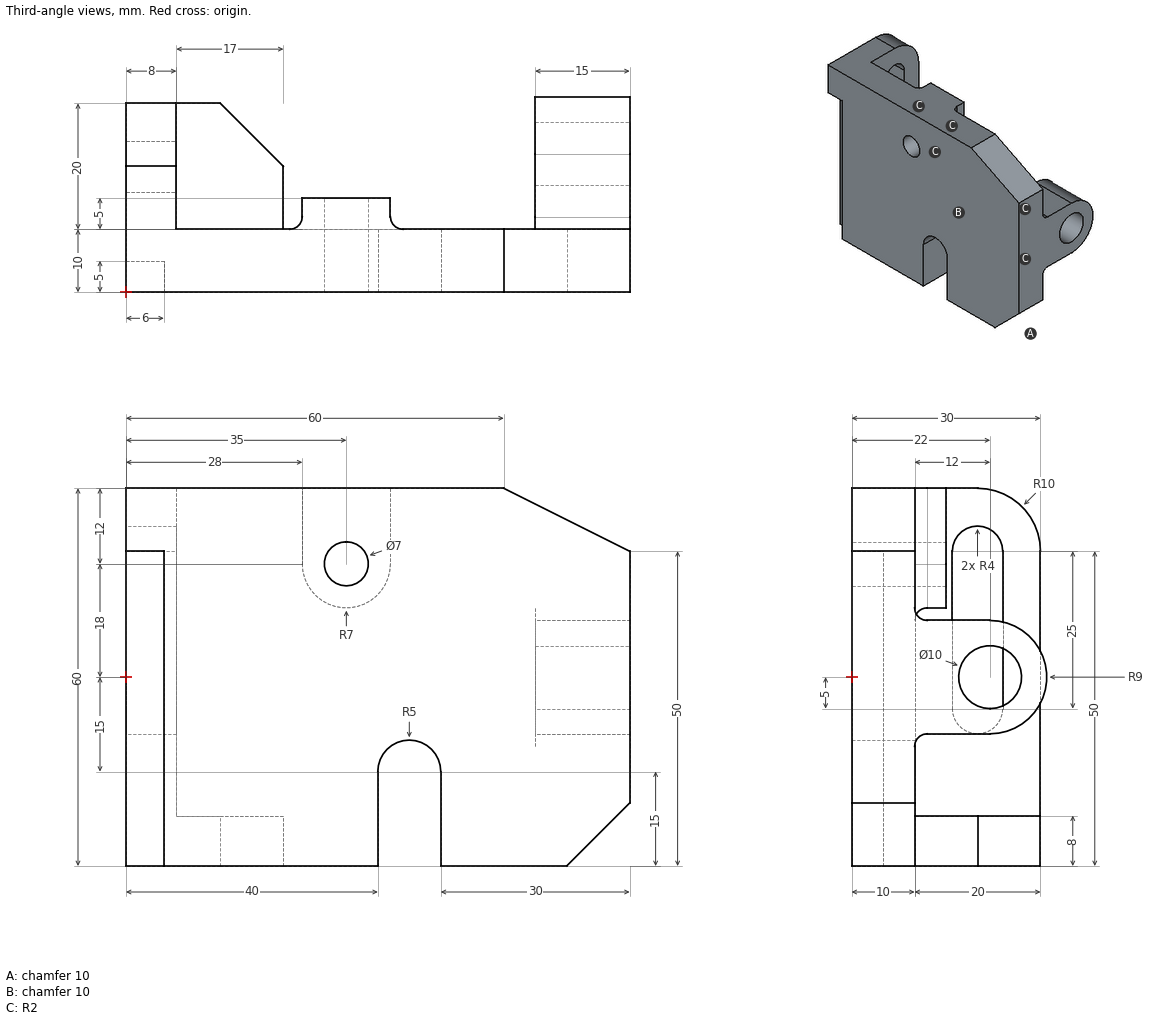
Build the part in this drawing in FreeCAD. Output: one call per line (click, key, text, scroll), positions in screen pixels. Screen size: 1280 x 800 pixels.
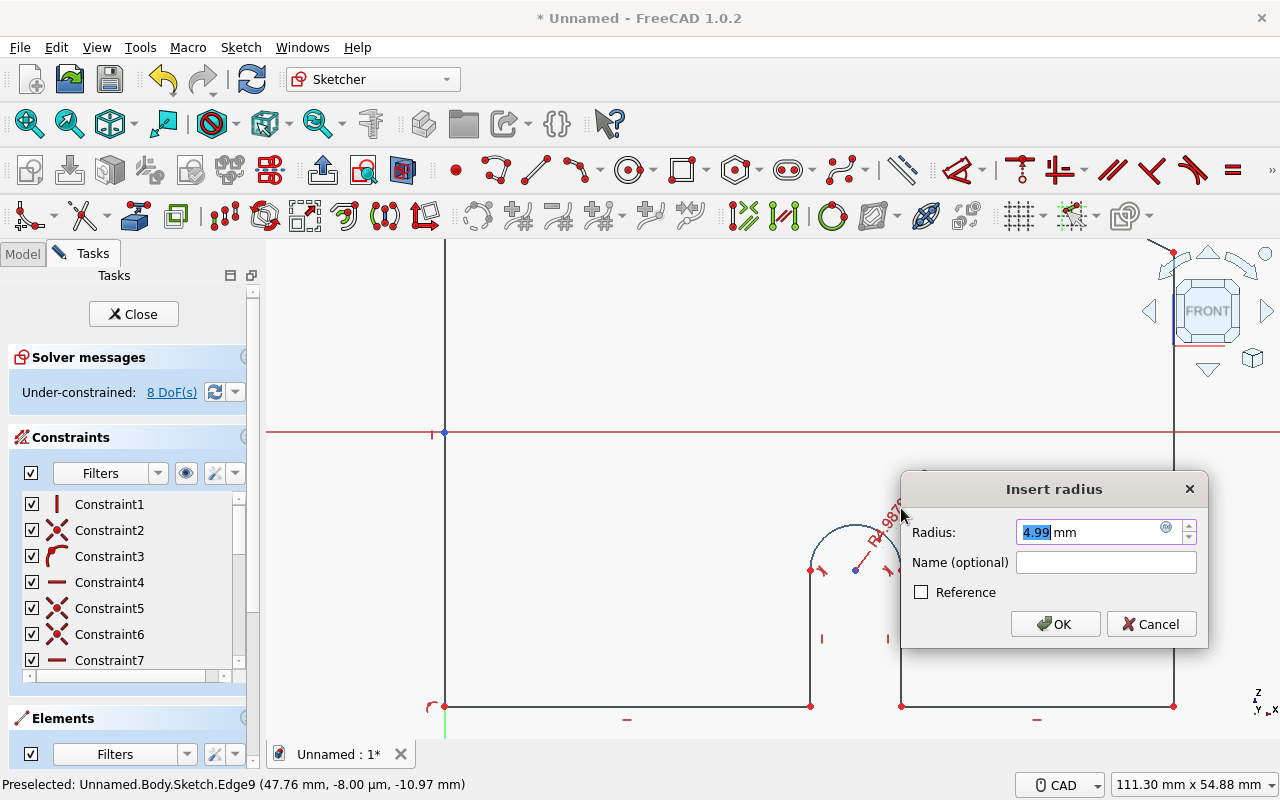
text(5)
key(Return)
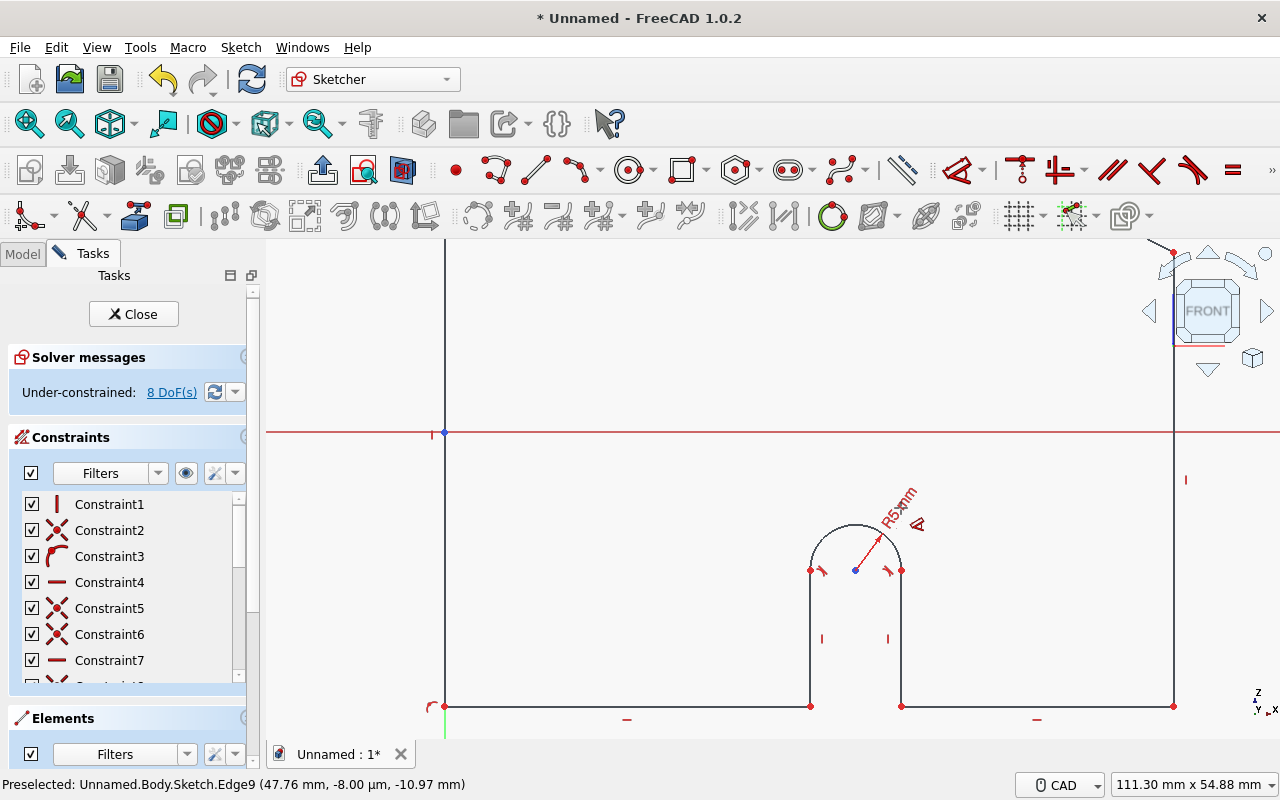
click(810, 611)
click(844, 639)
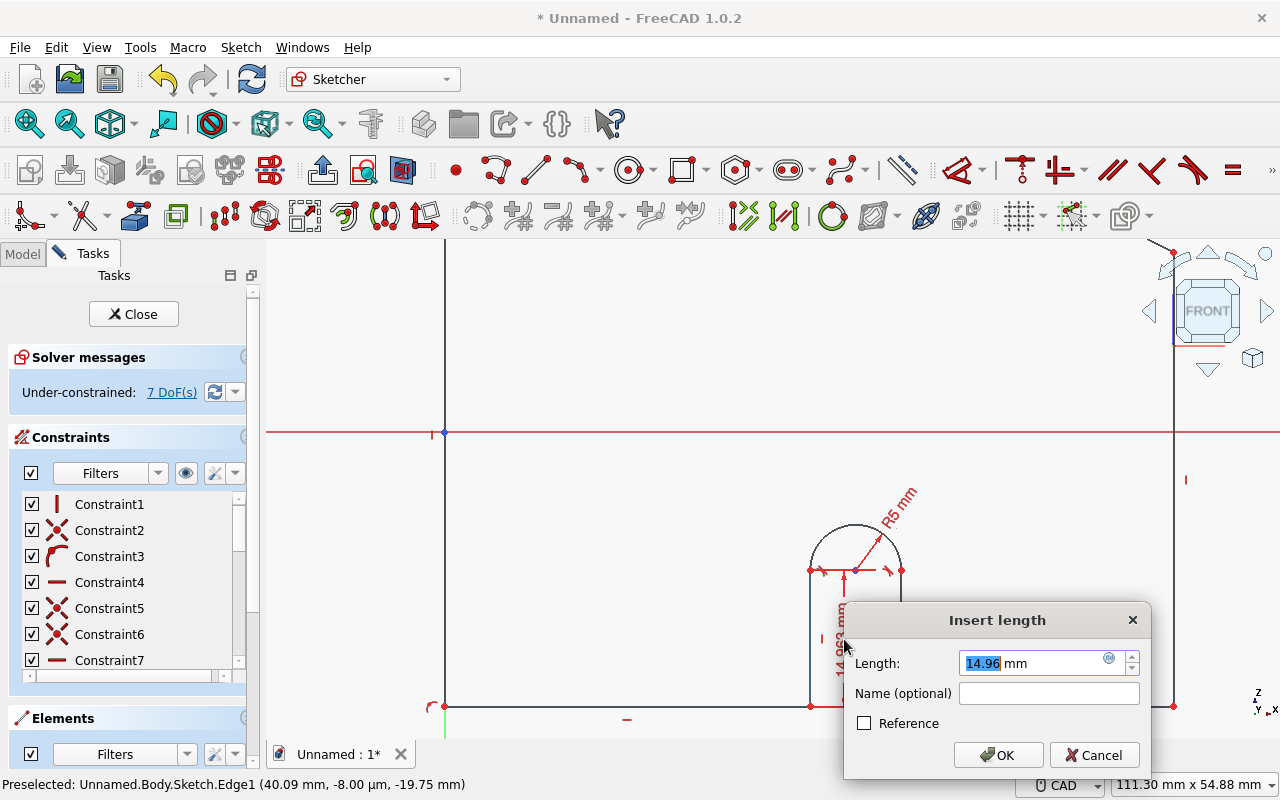
text(15)
key(Return)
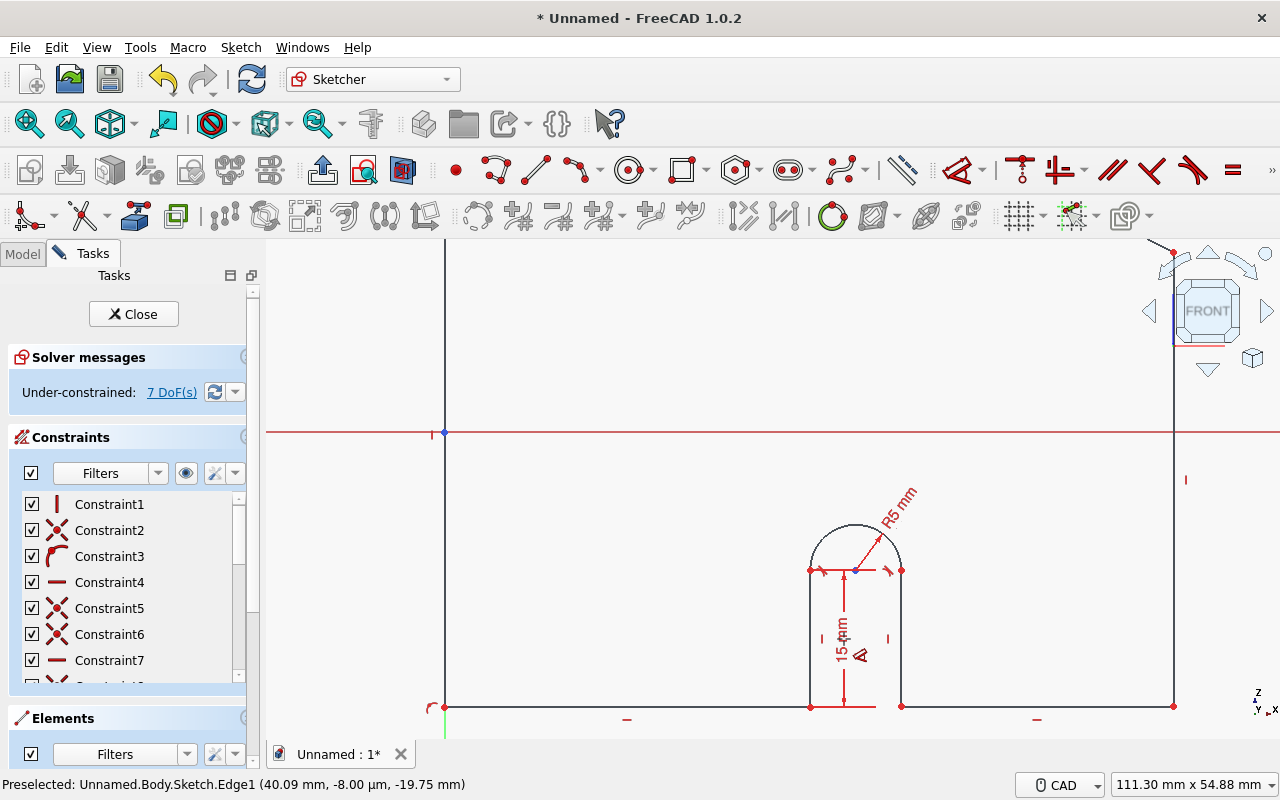
click(701, 707)
click(628, 673)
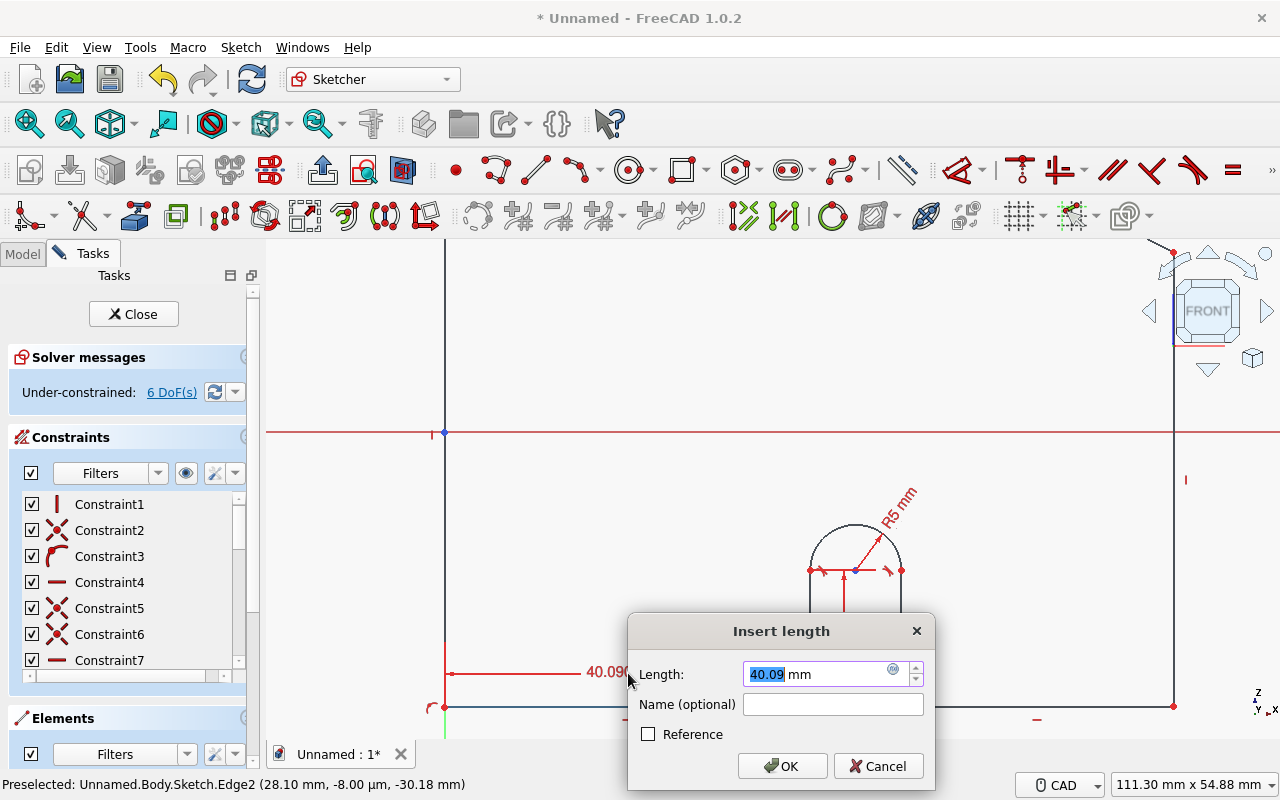
text(40)
key(Return)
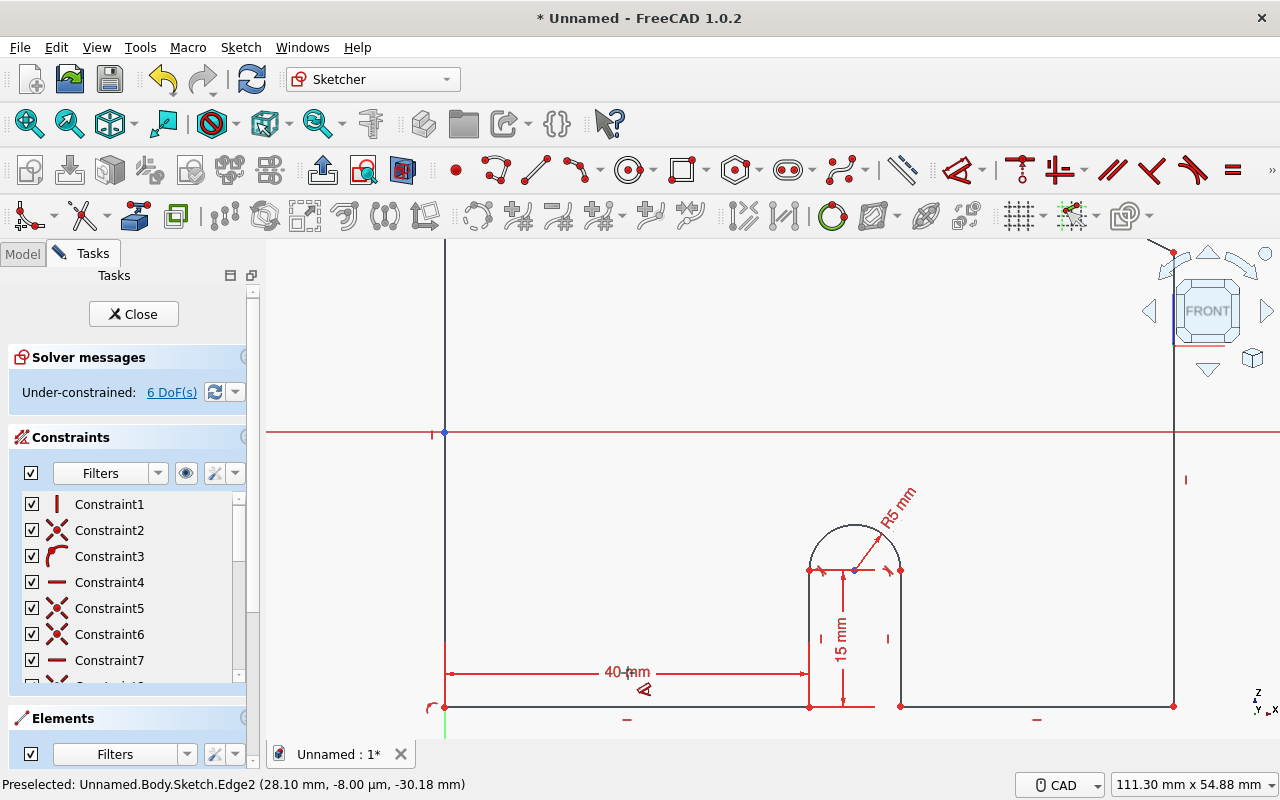
click(445, 543)
click(411, 487)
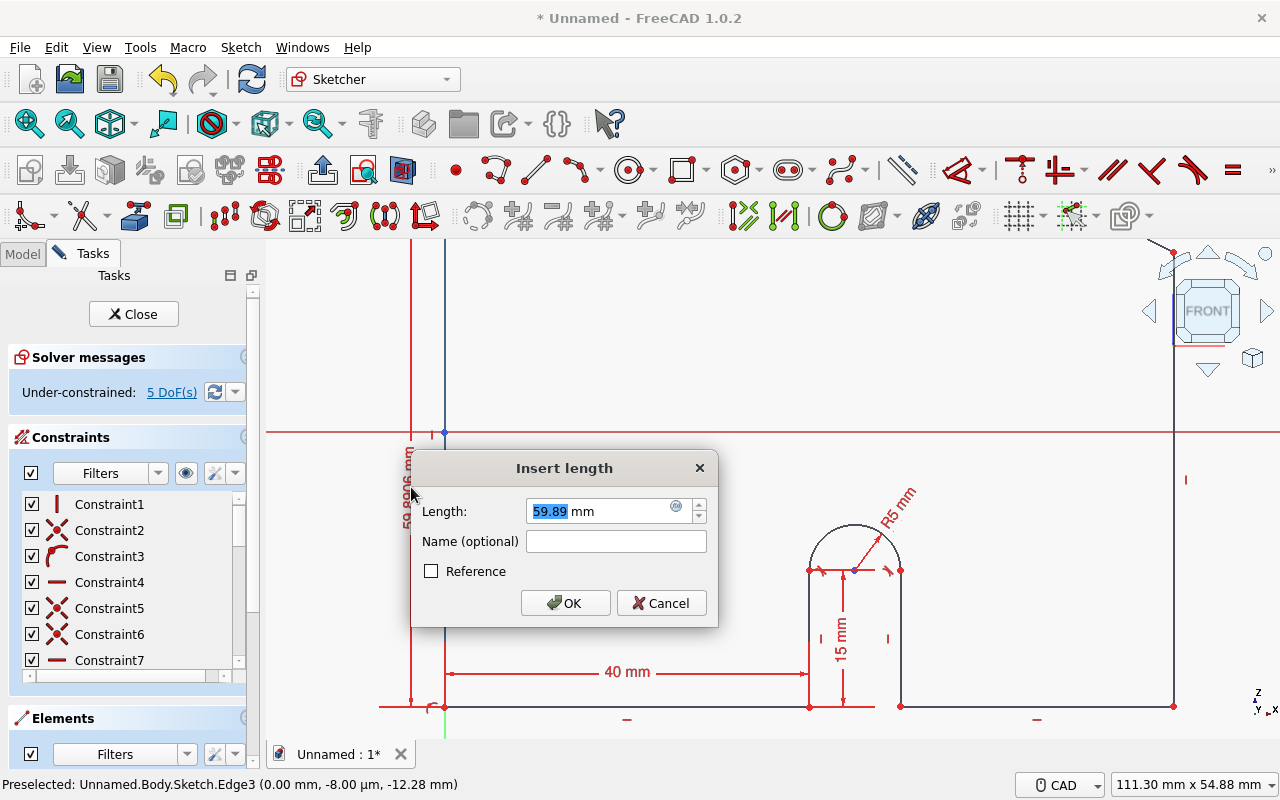
text(60)
key(Return)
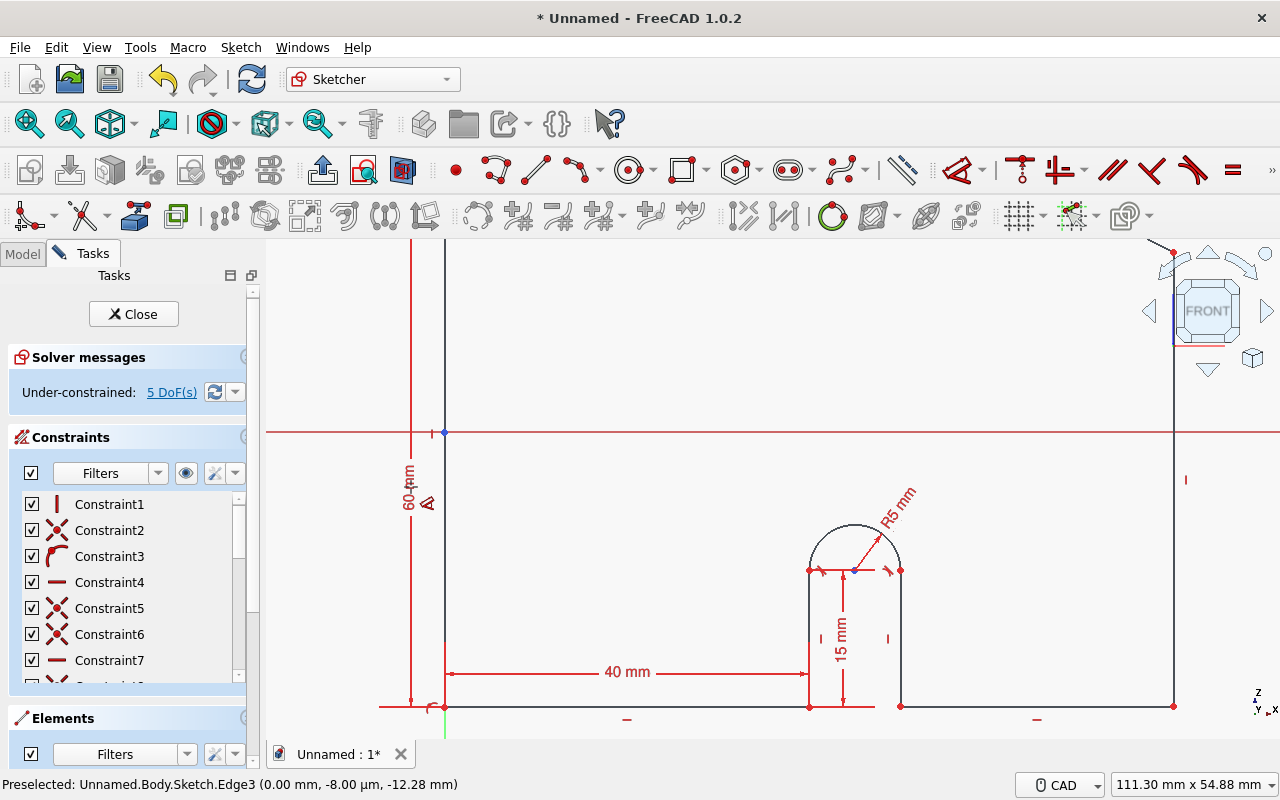
scroll(577, 558, down, 3)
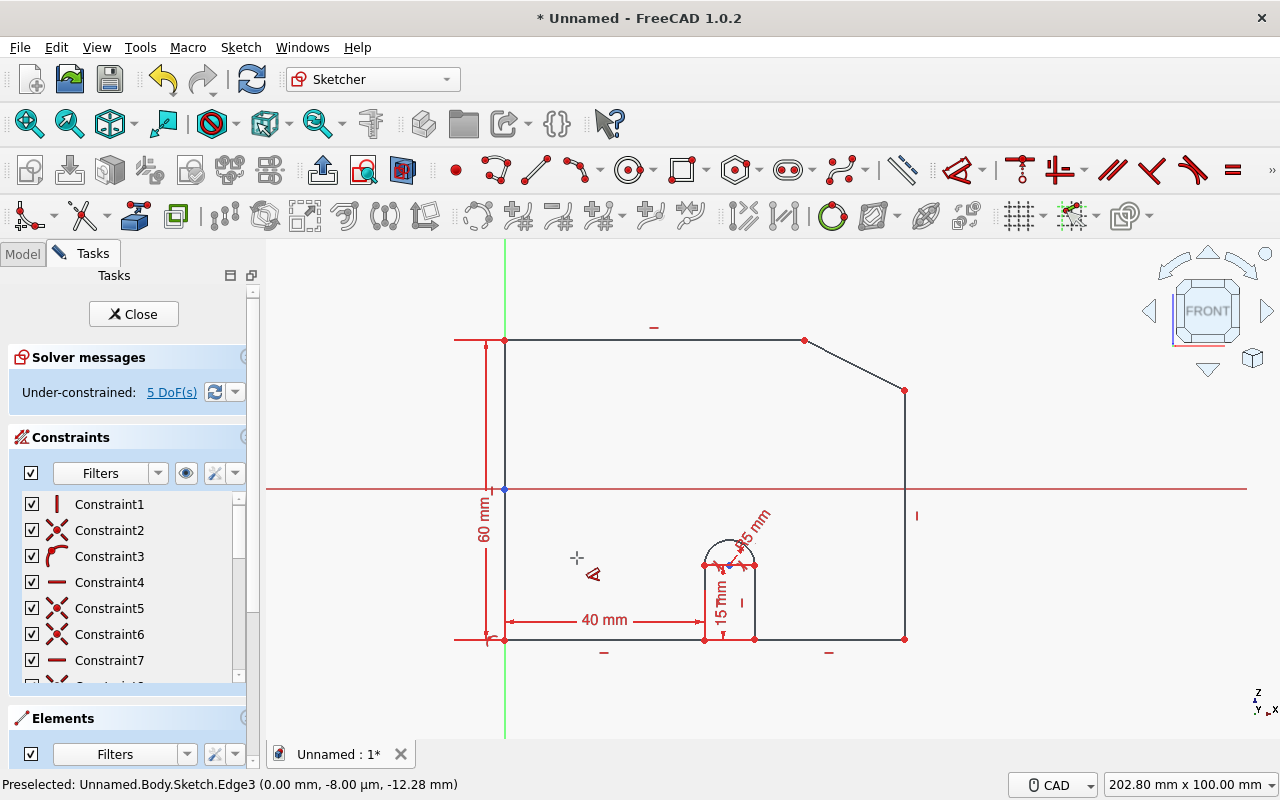
click(595, 340)
click(655, 306)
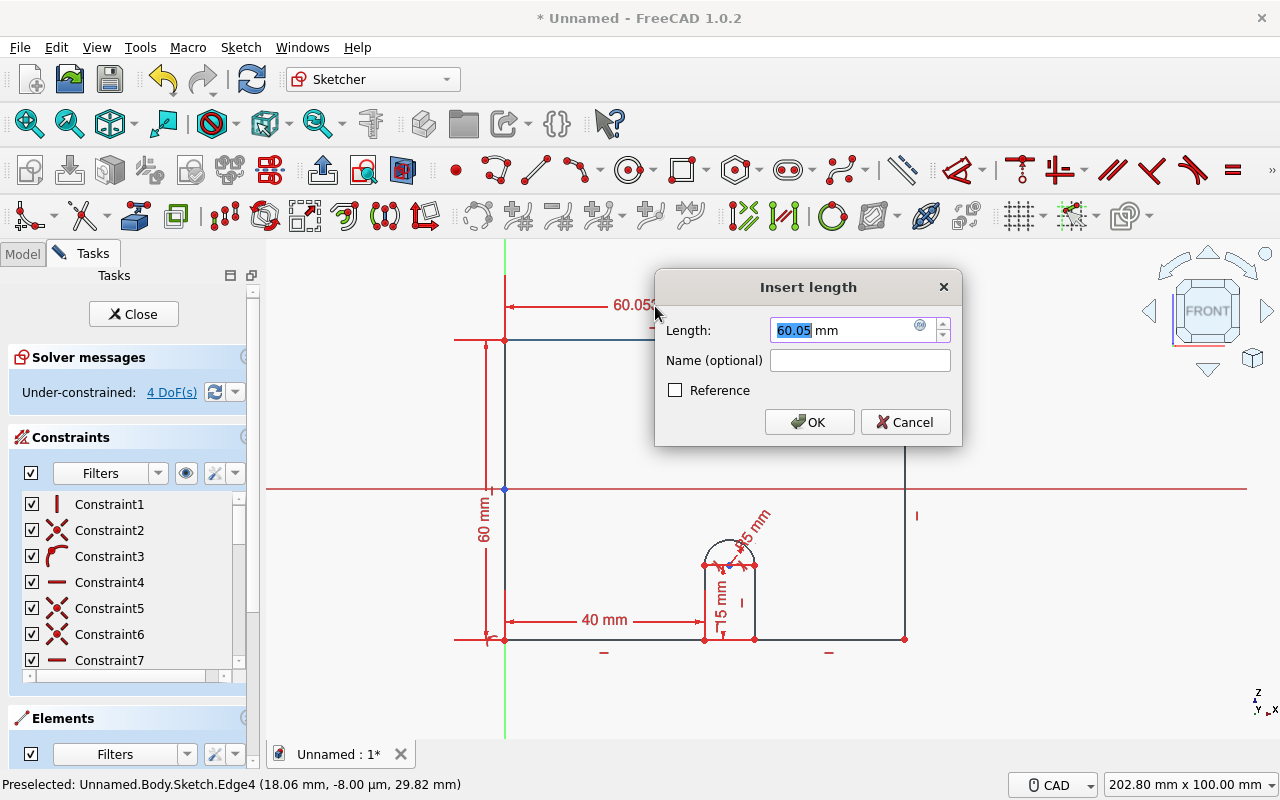
text(60)
key(Return)